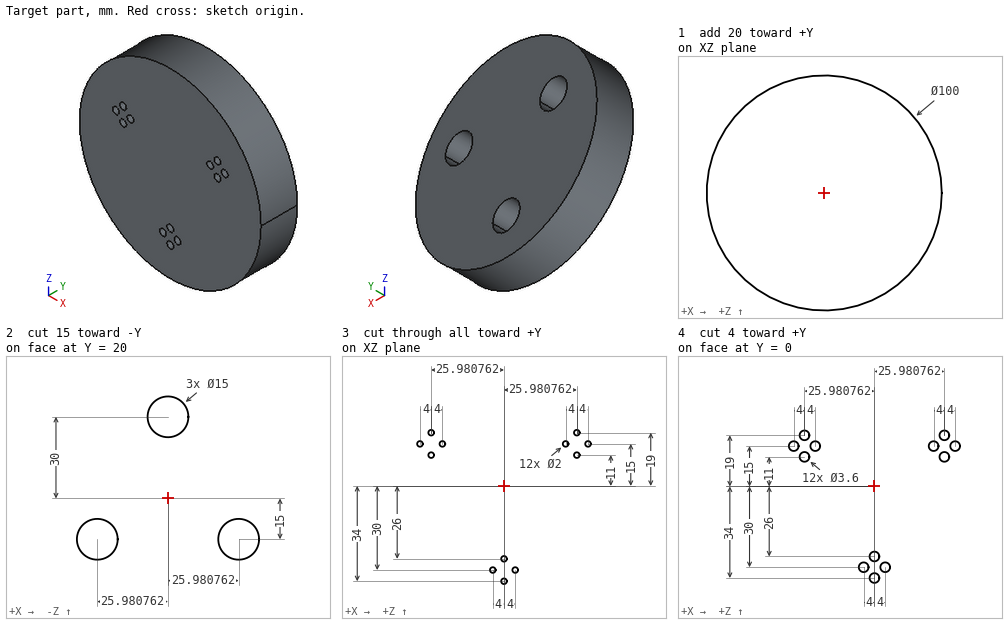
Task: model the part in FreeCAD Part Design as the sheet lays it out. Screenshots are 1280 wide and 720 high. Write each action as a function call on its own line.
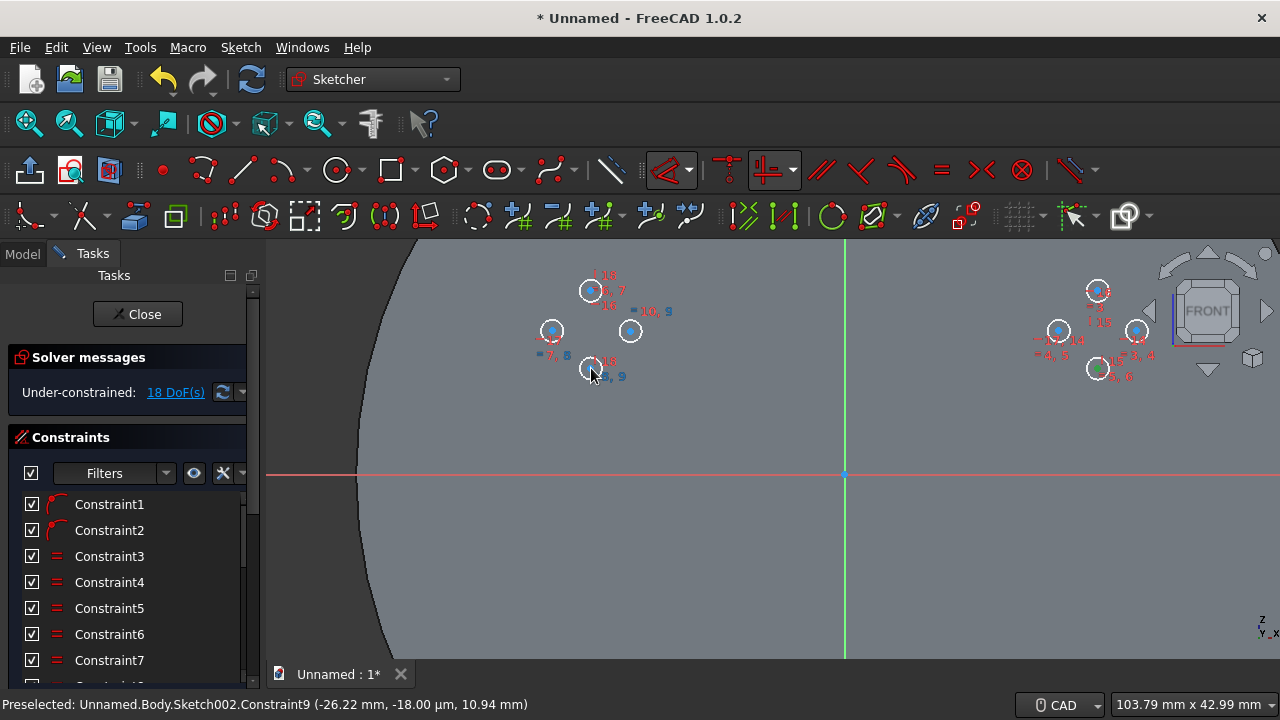
click(589, 371)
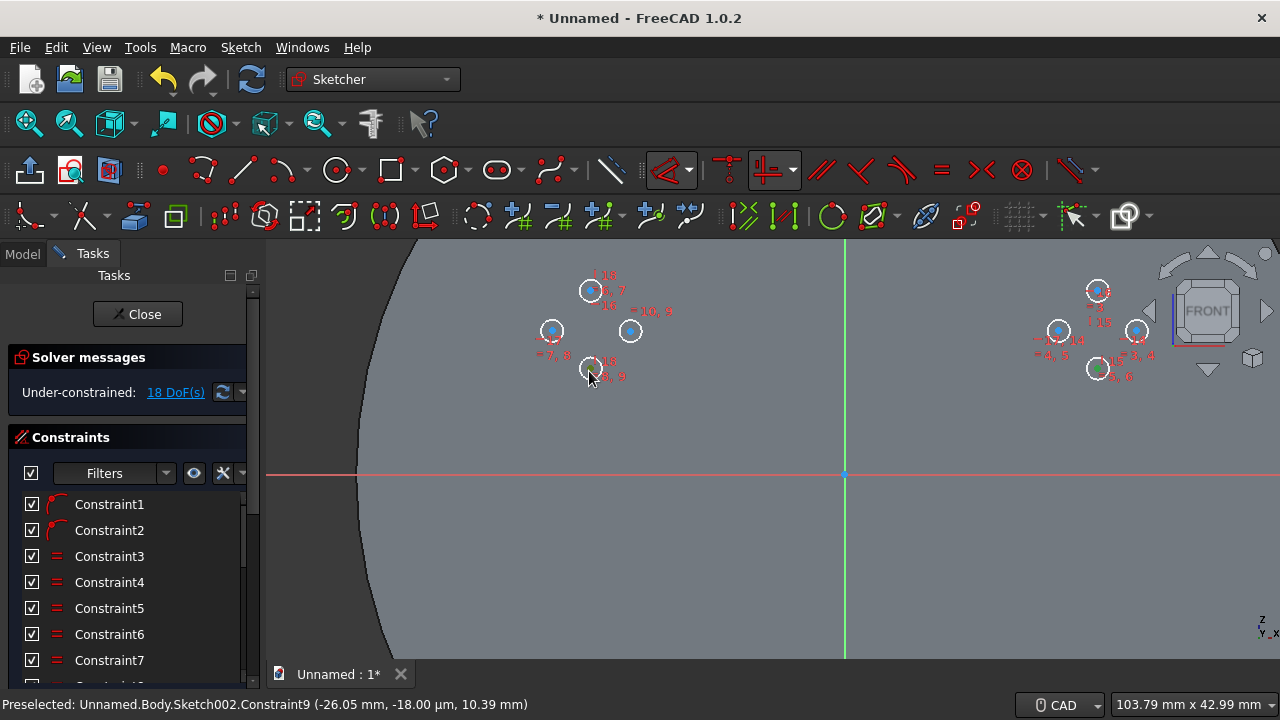
key(h)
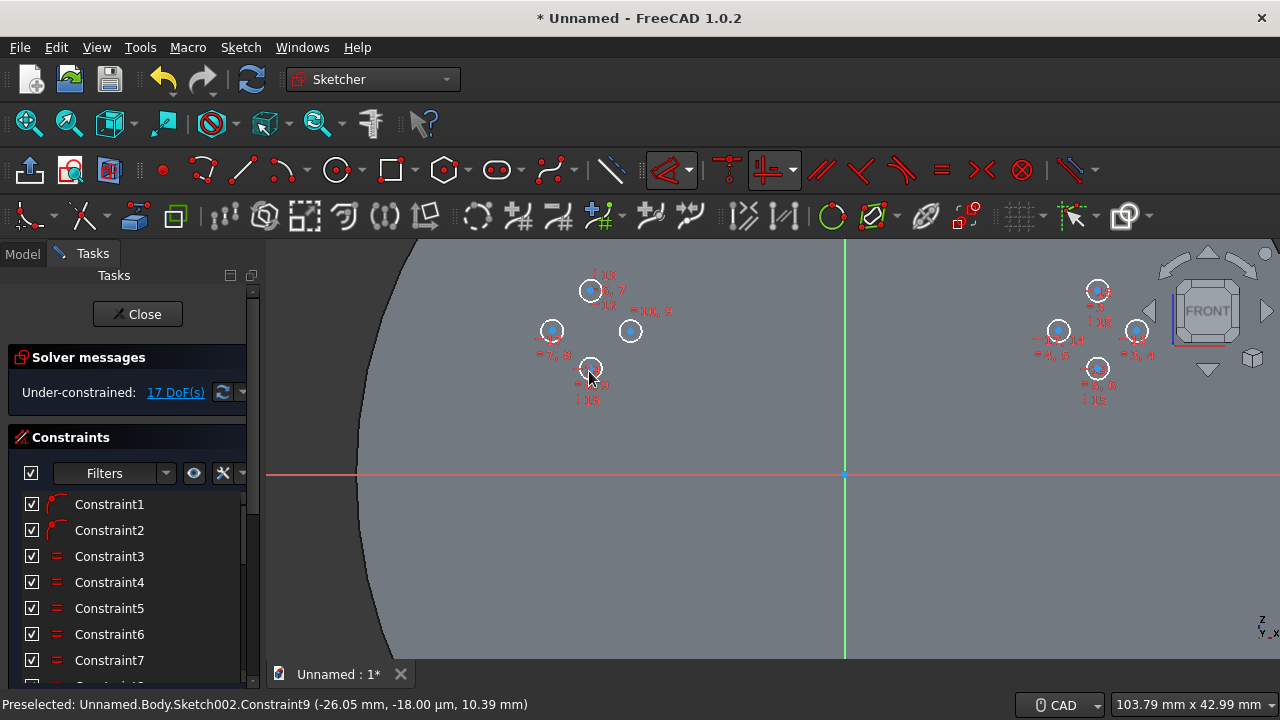
click(552, 331)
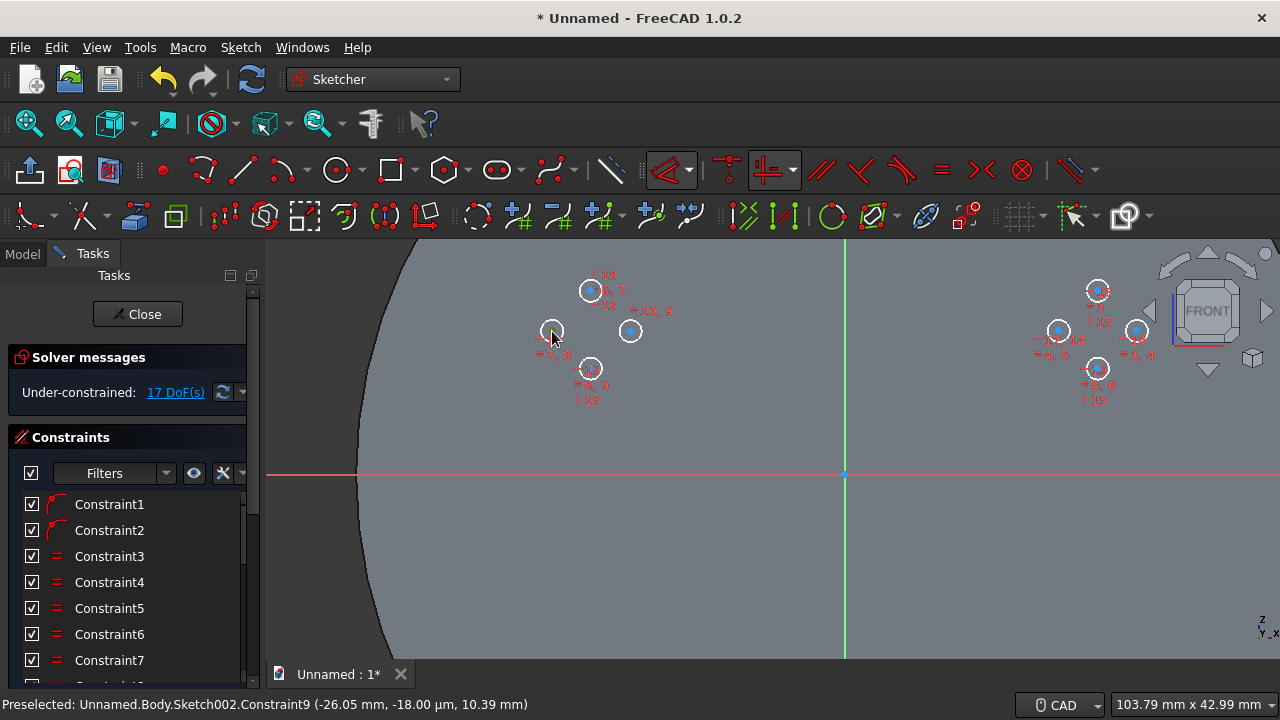
click(631, 331)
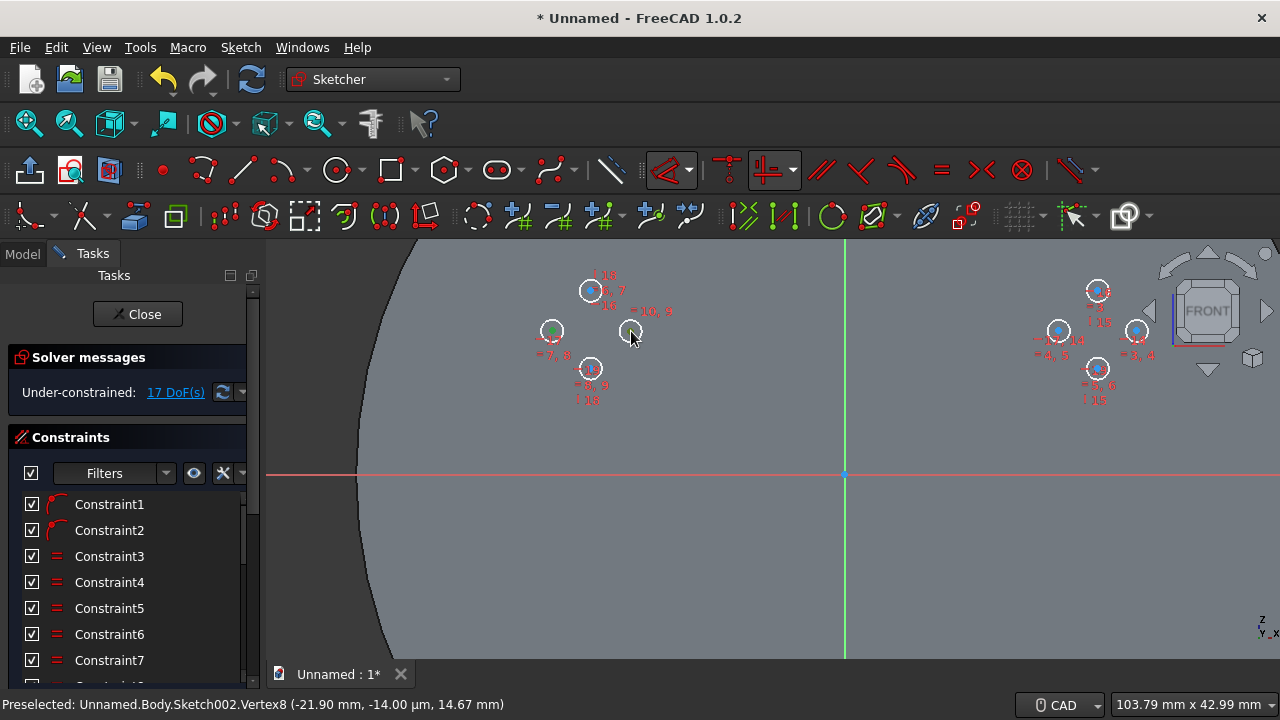
key(h)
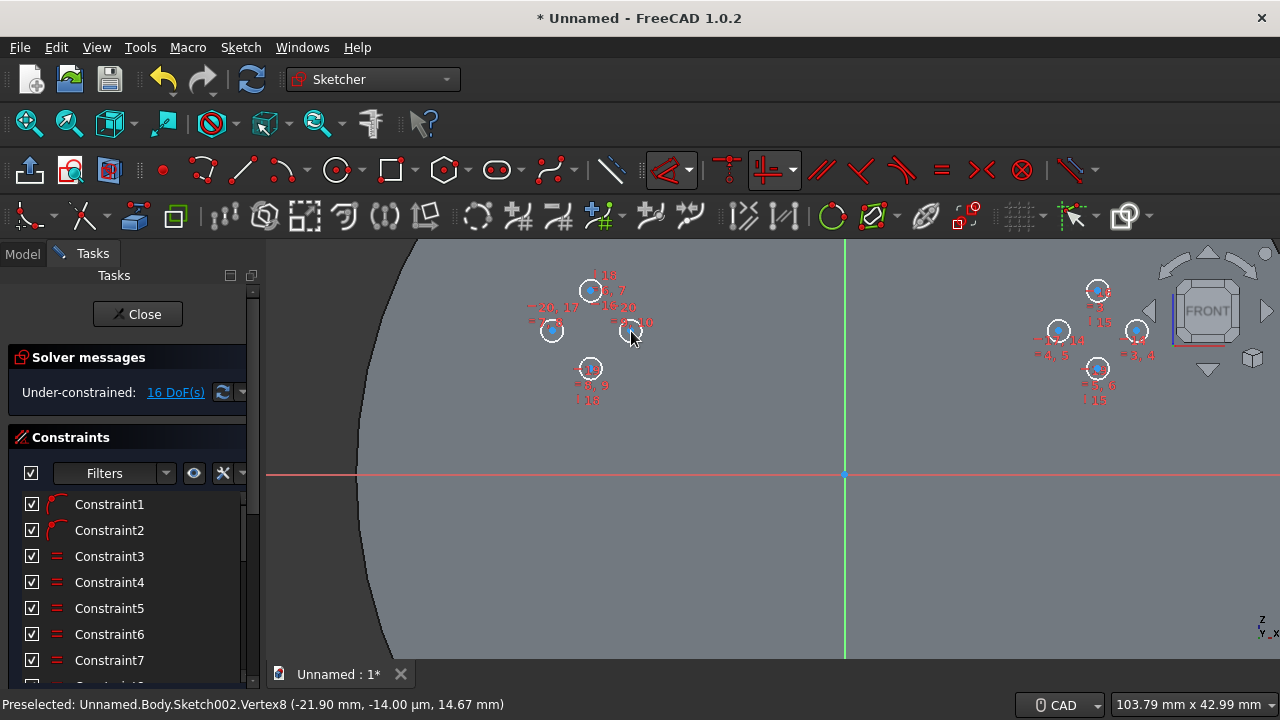
scroll(590, 368, down, 4)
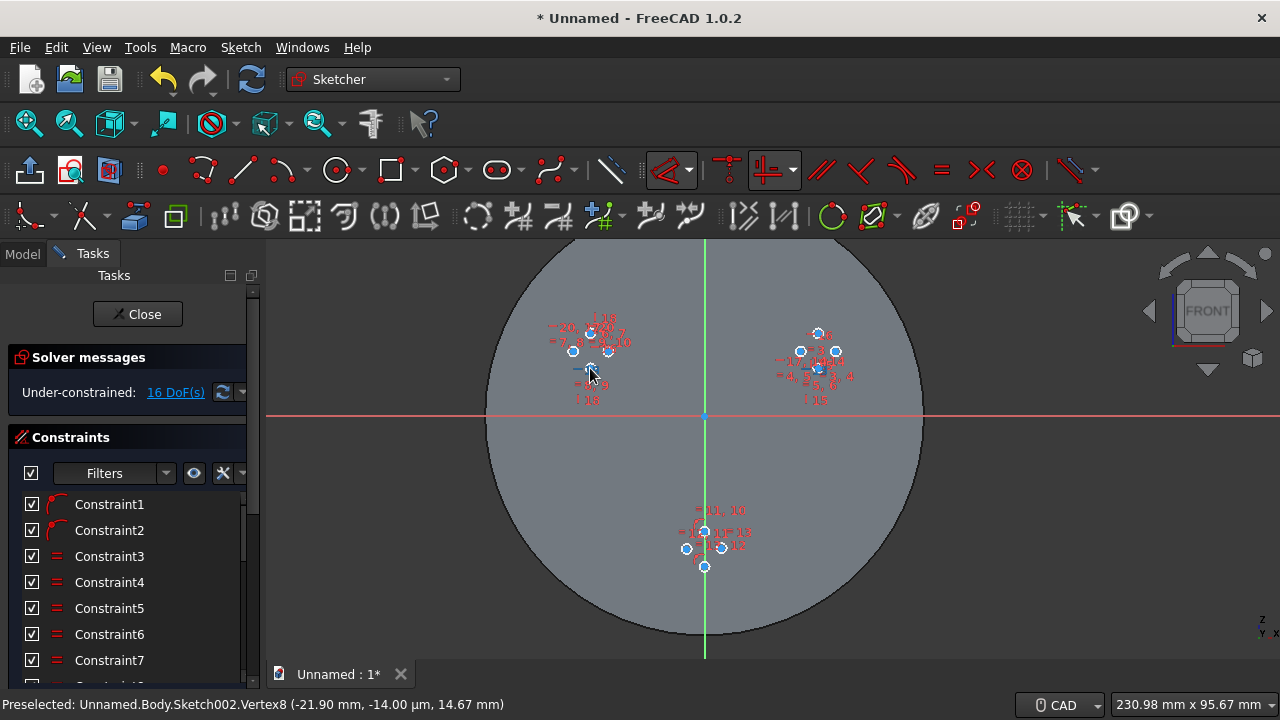
click(687, 549)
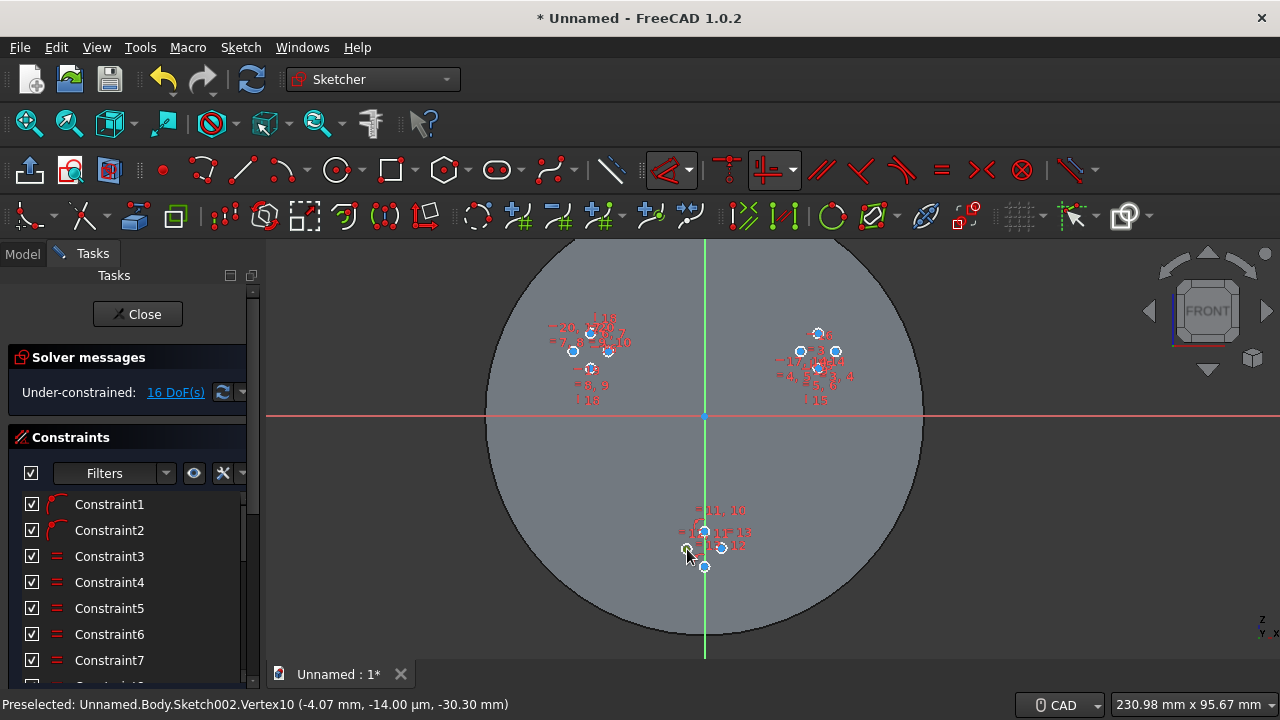
click(722, 548)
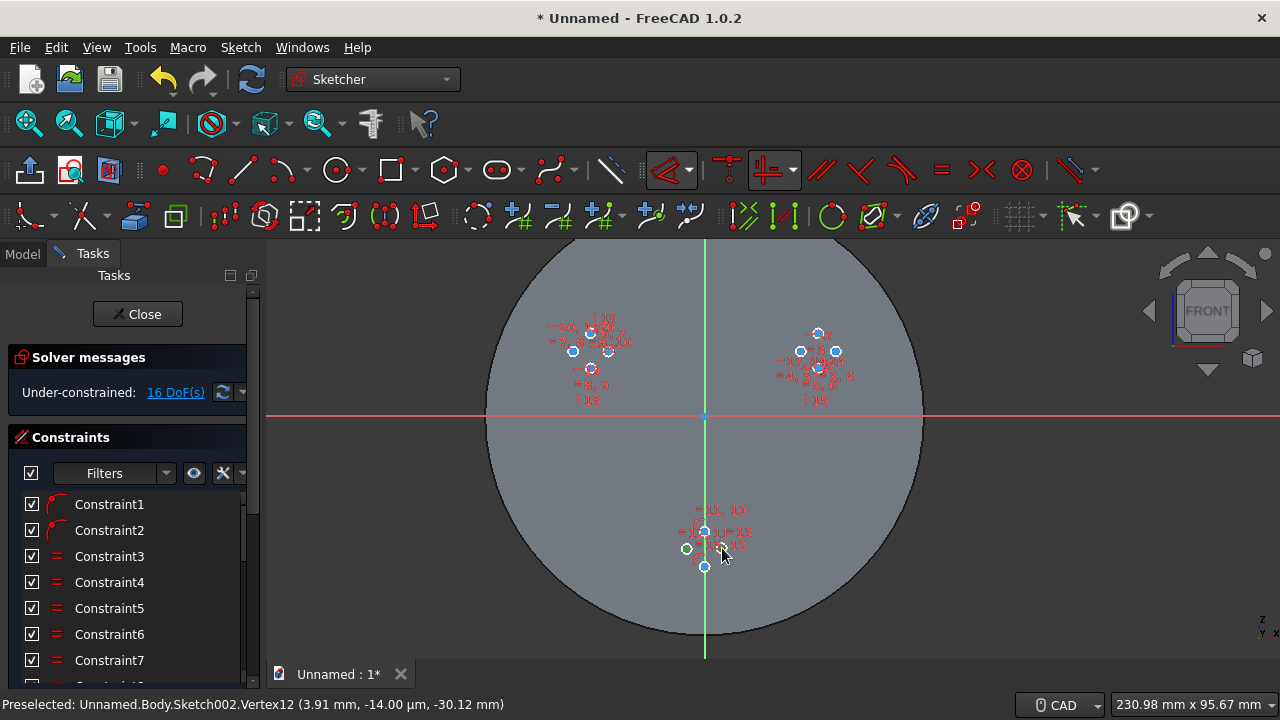
key(h)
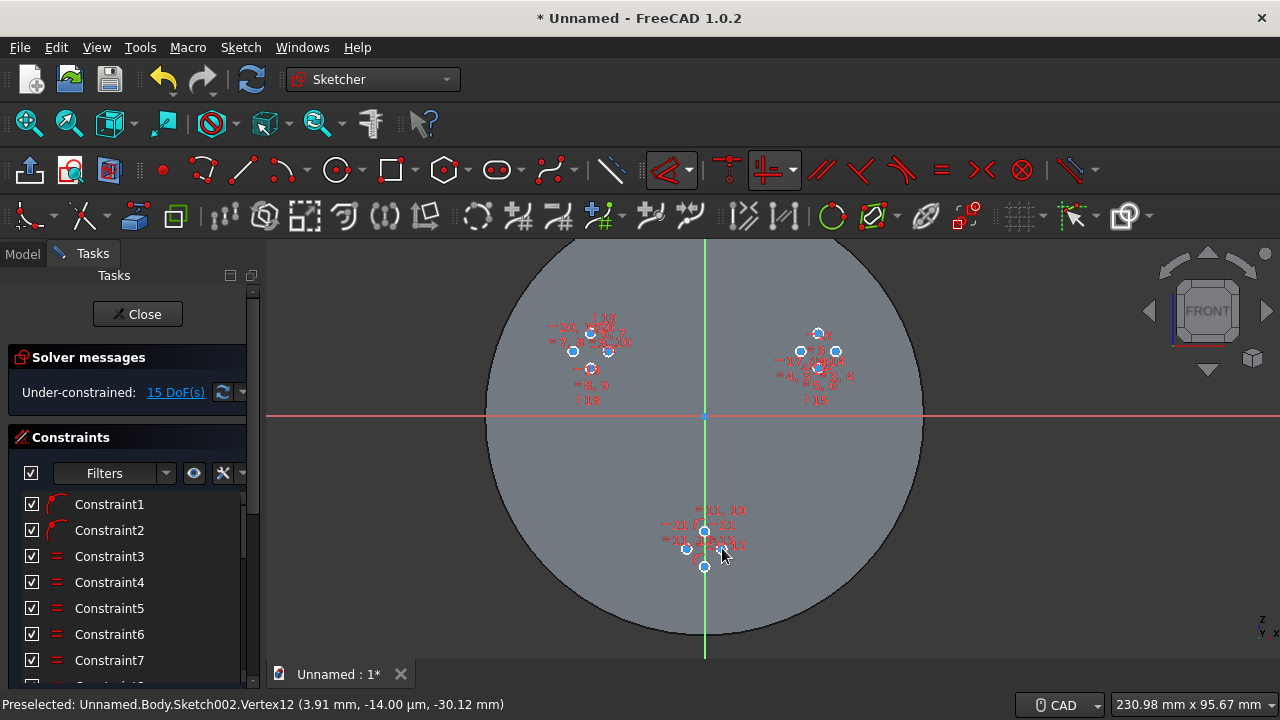
scroll(822, 330, up, 8)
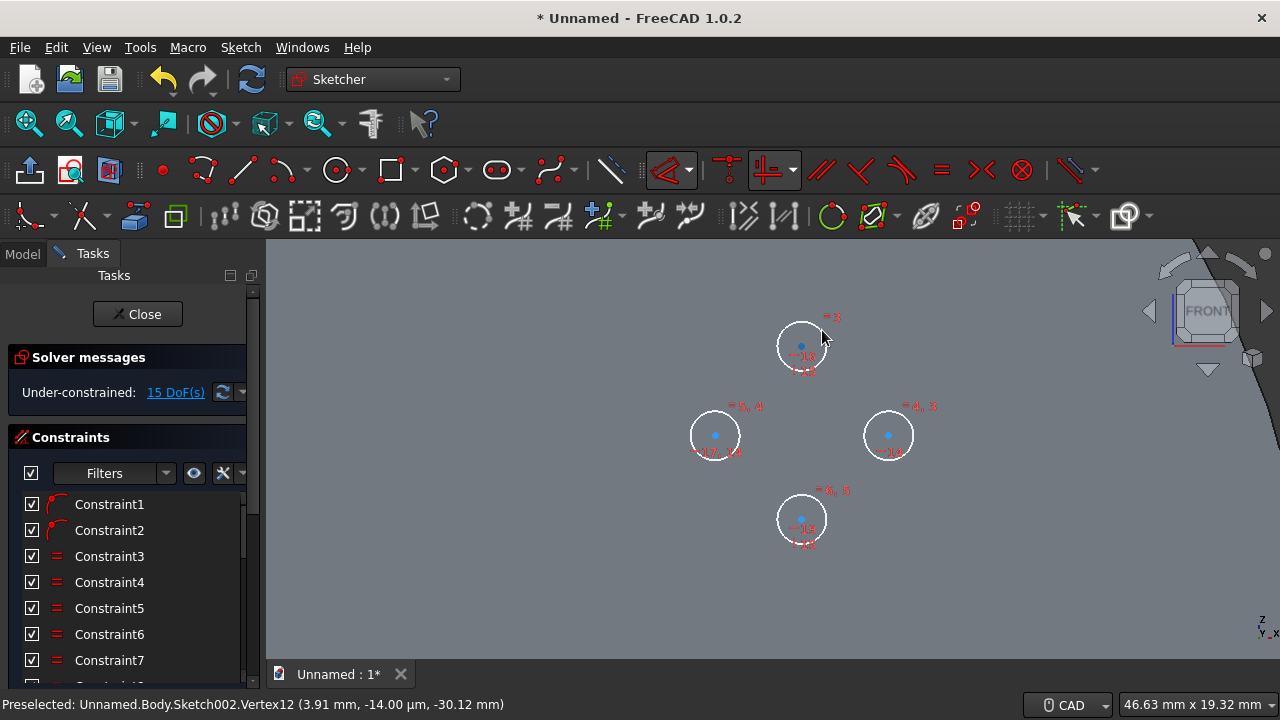
click(819, 329)